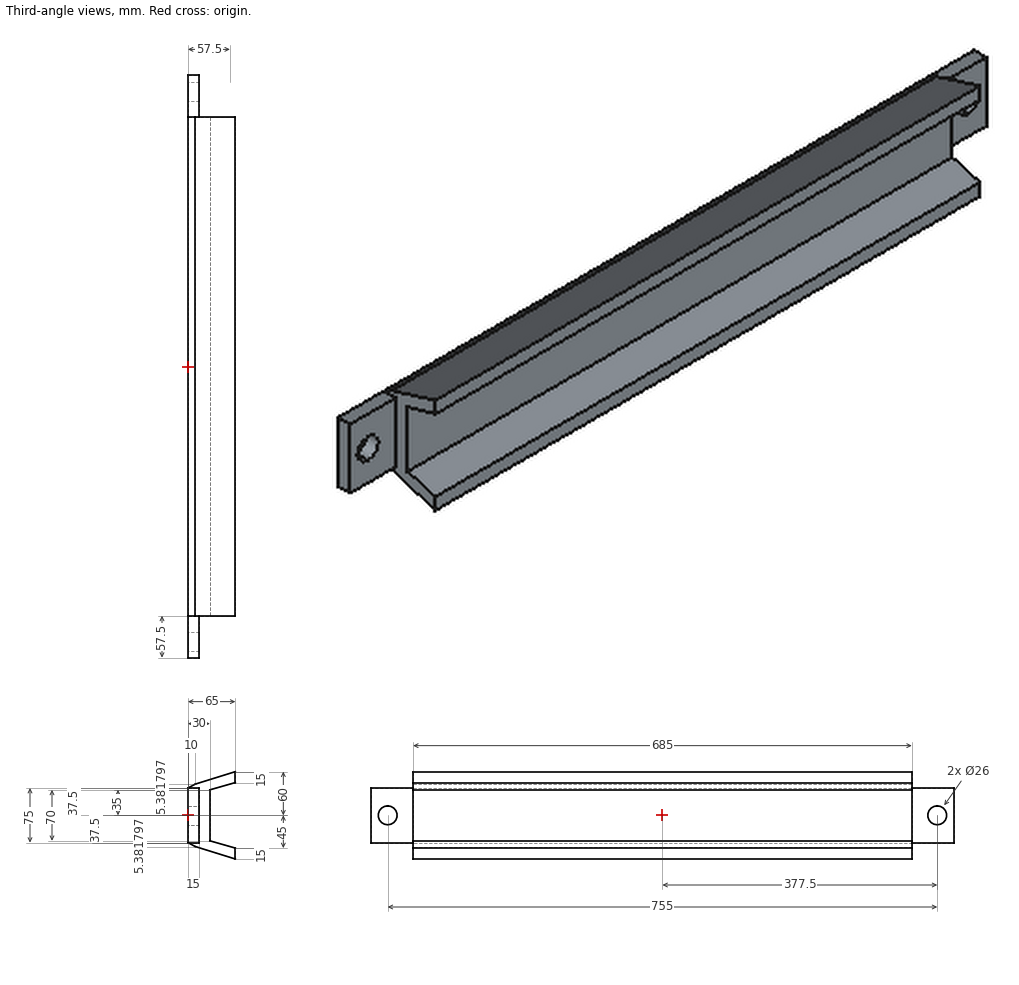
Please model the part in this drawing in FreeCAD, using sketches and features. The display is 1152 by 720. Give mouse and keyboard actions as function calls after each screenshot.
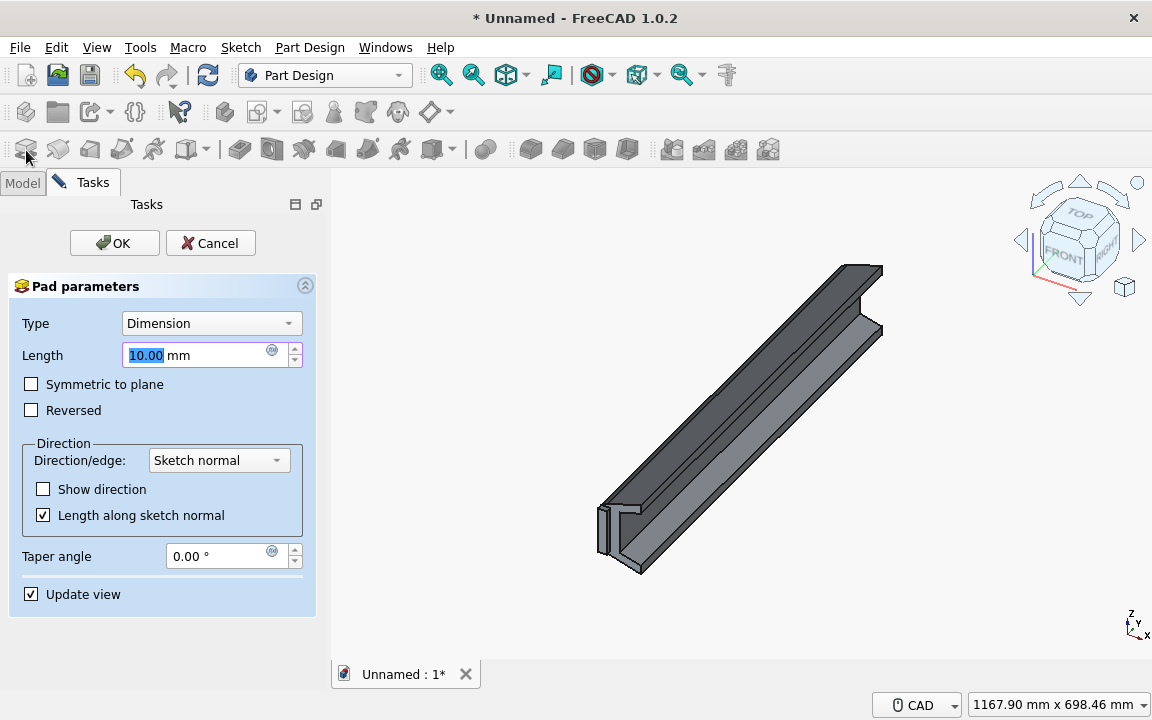
text(57.5)
key(Tab)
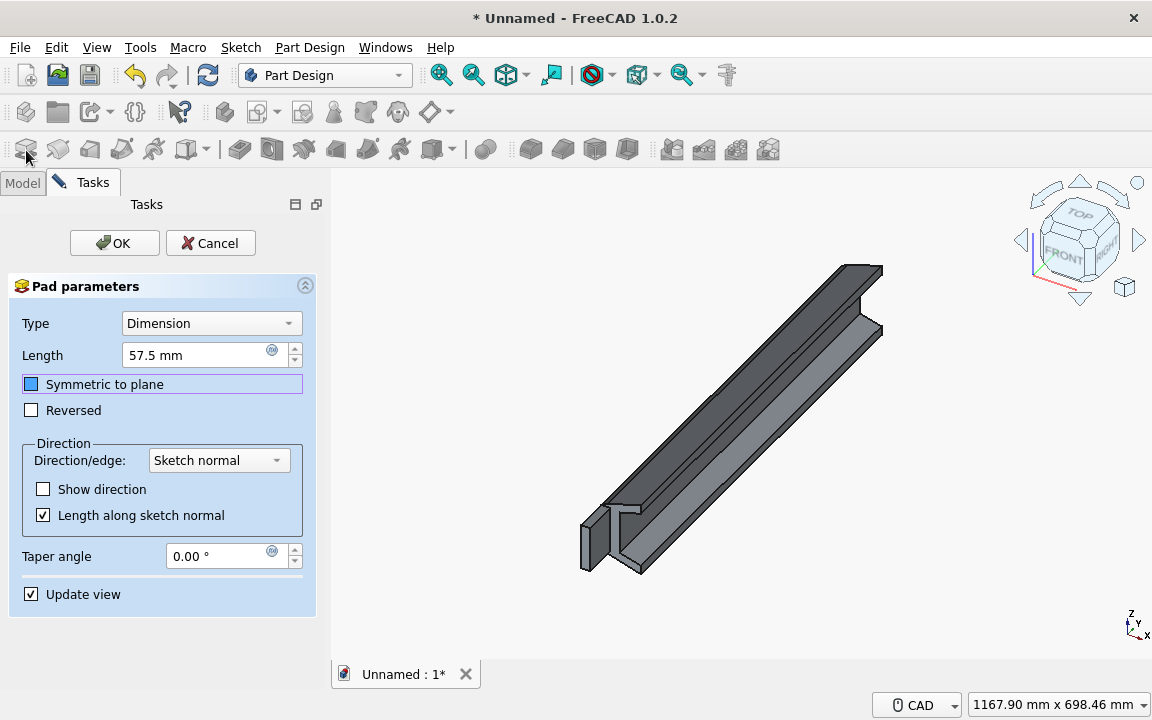
click(115, 243)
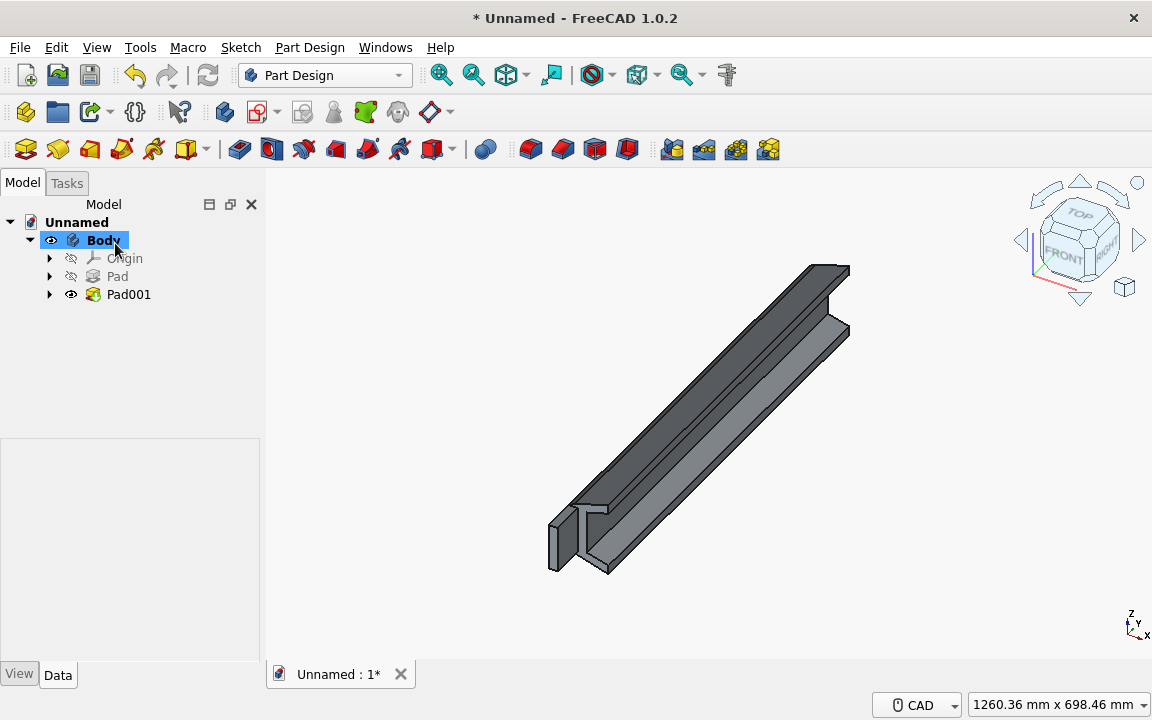
click(116, 294)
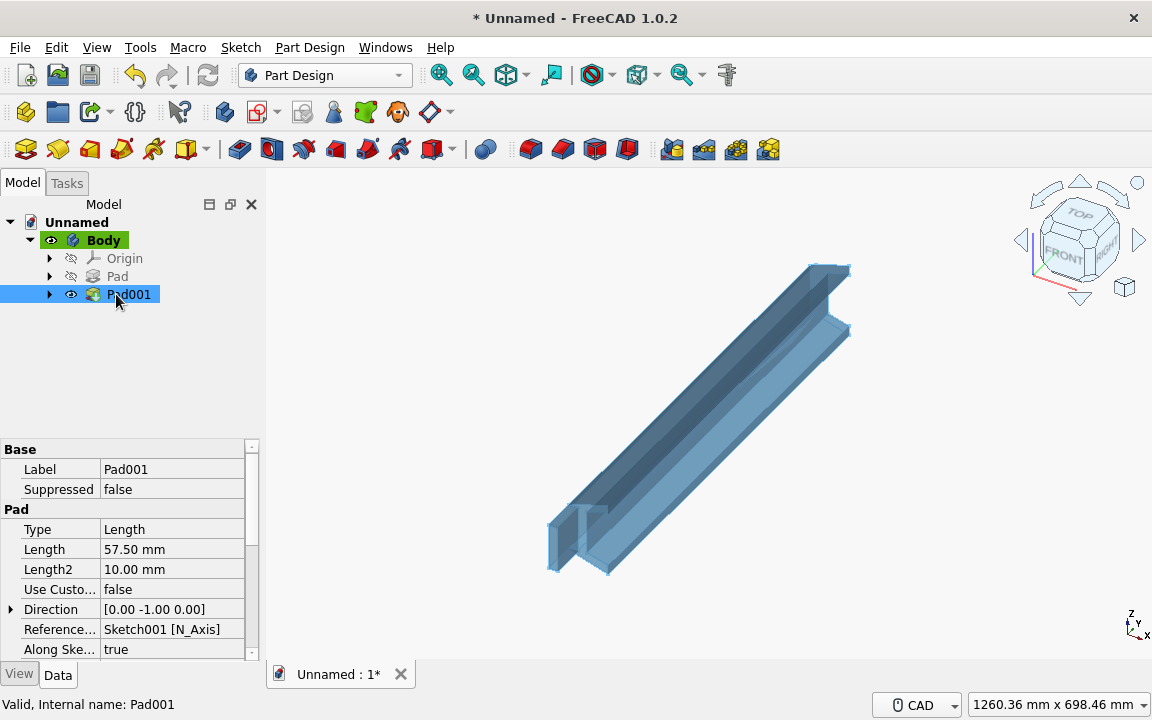
click(672, 150)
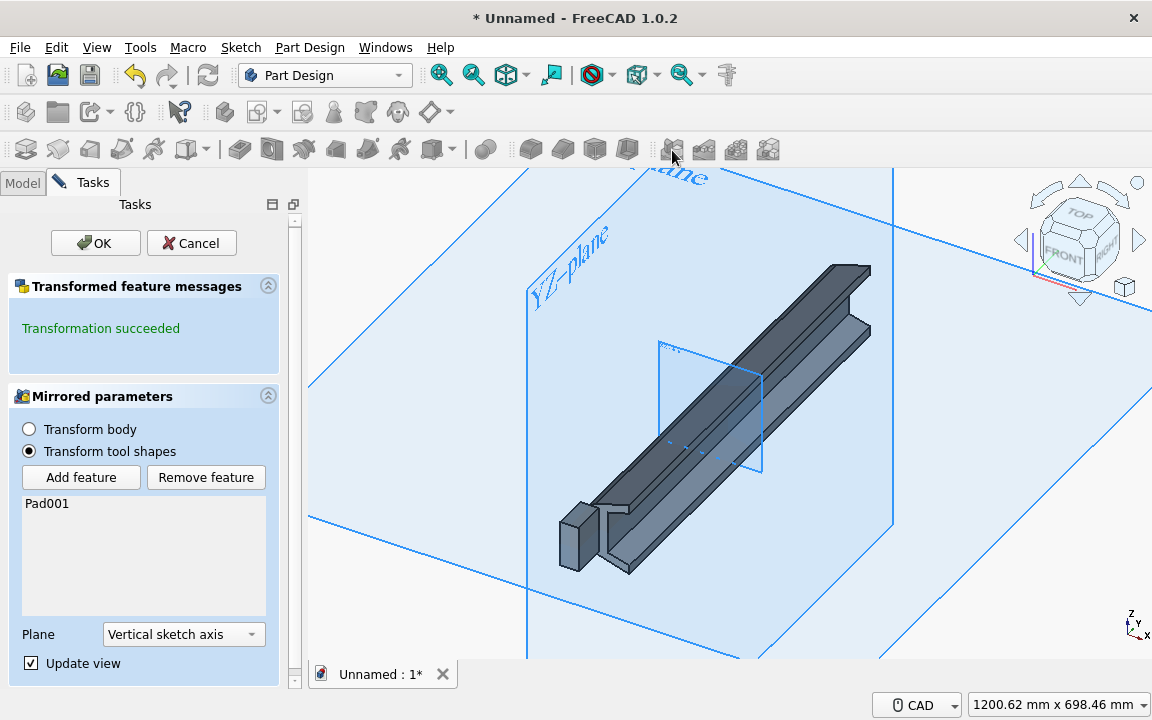
click(184, 634)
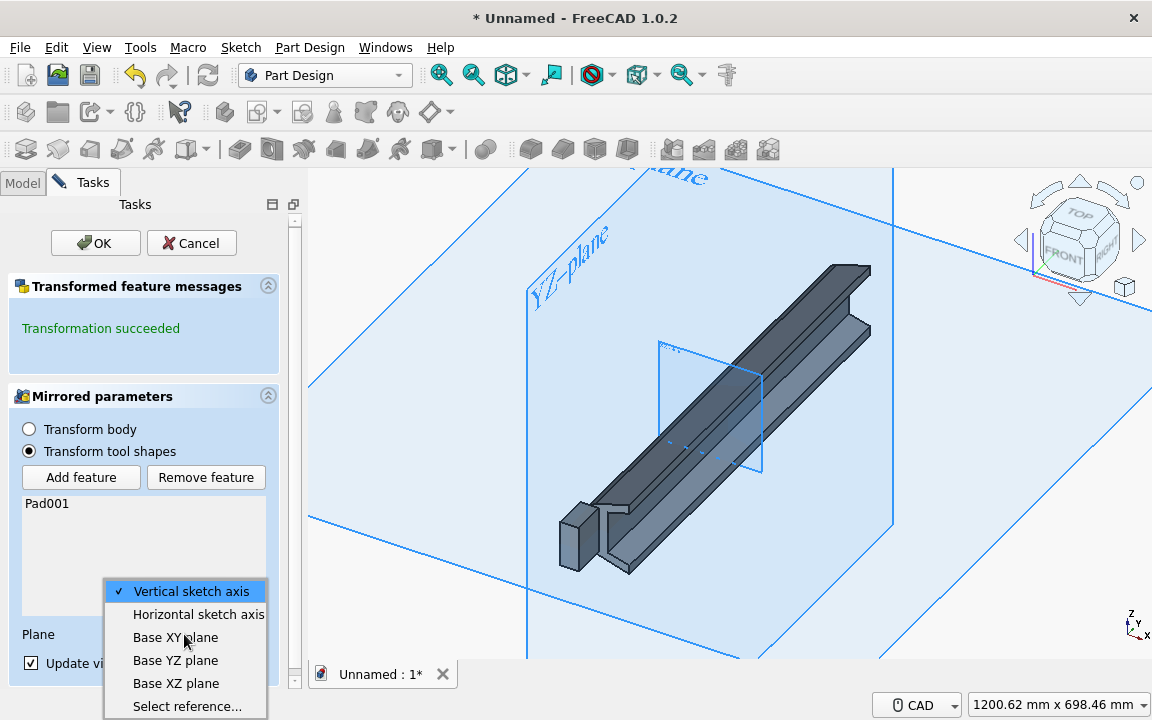
click(184, 684)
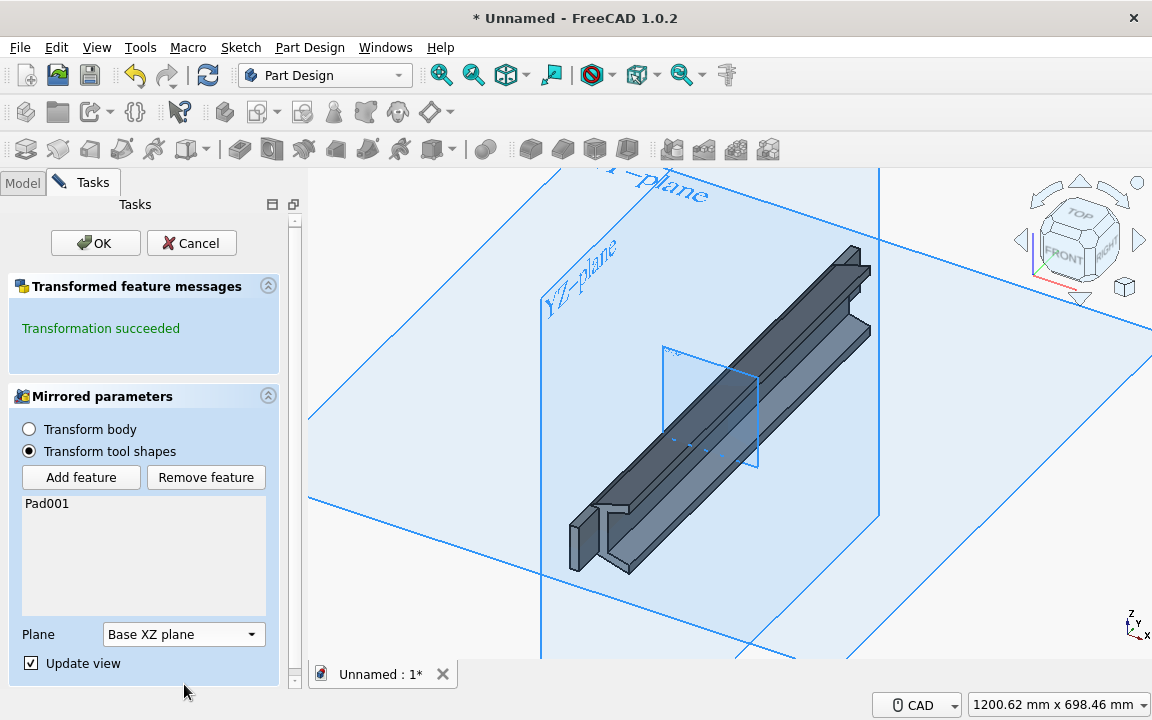
click(96, 243)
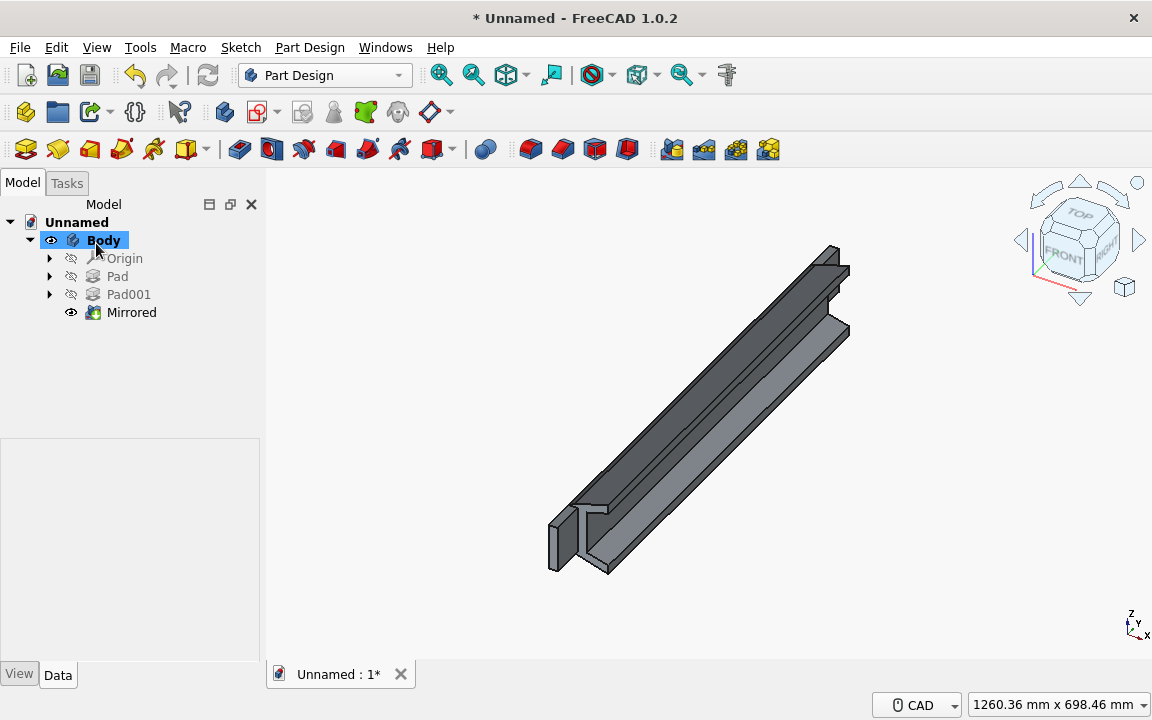
key(6)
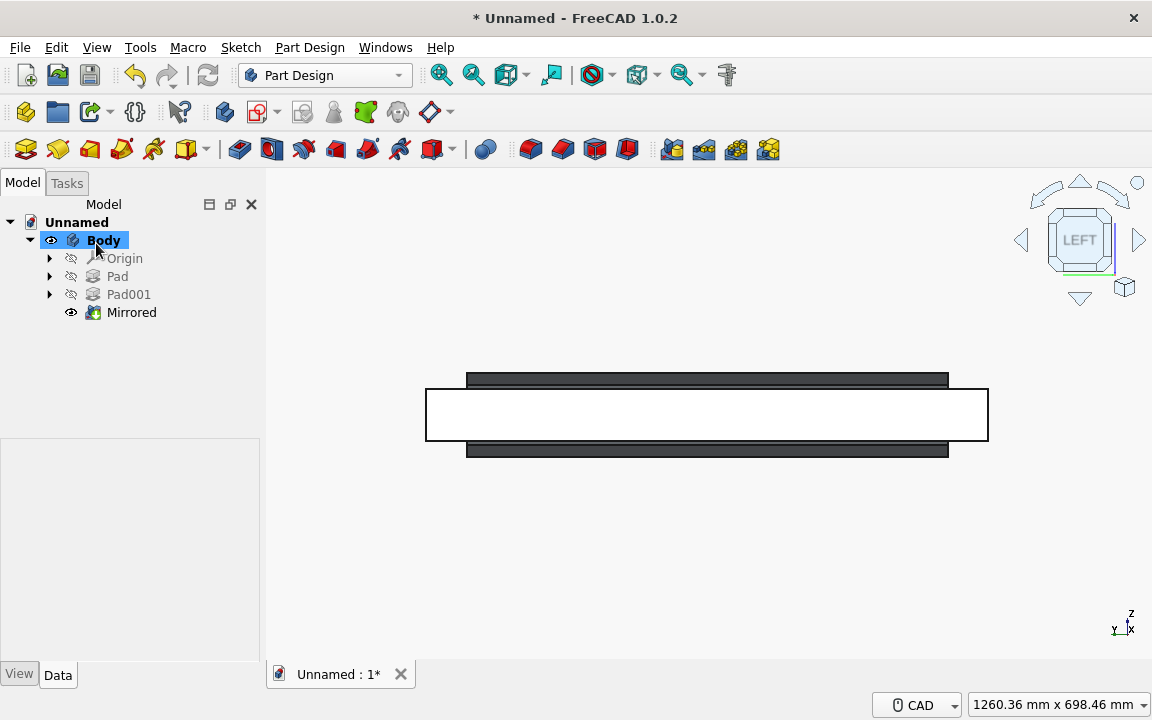
click(707, 414)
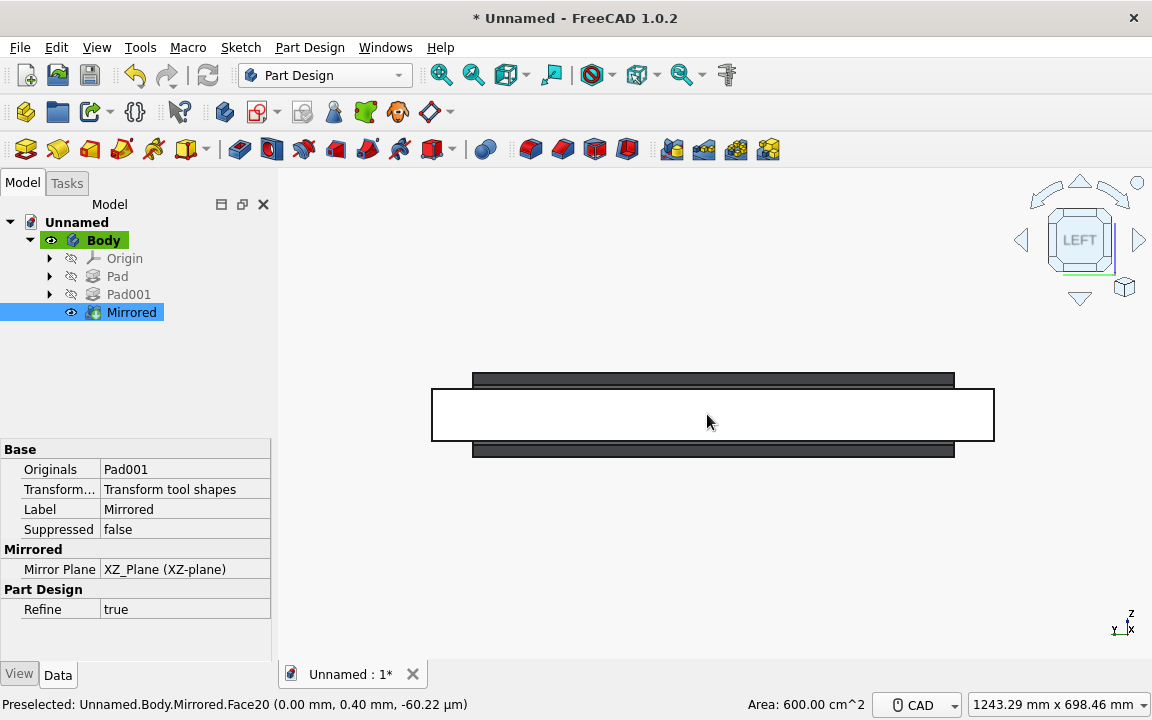
click(258, 112)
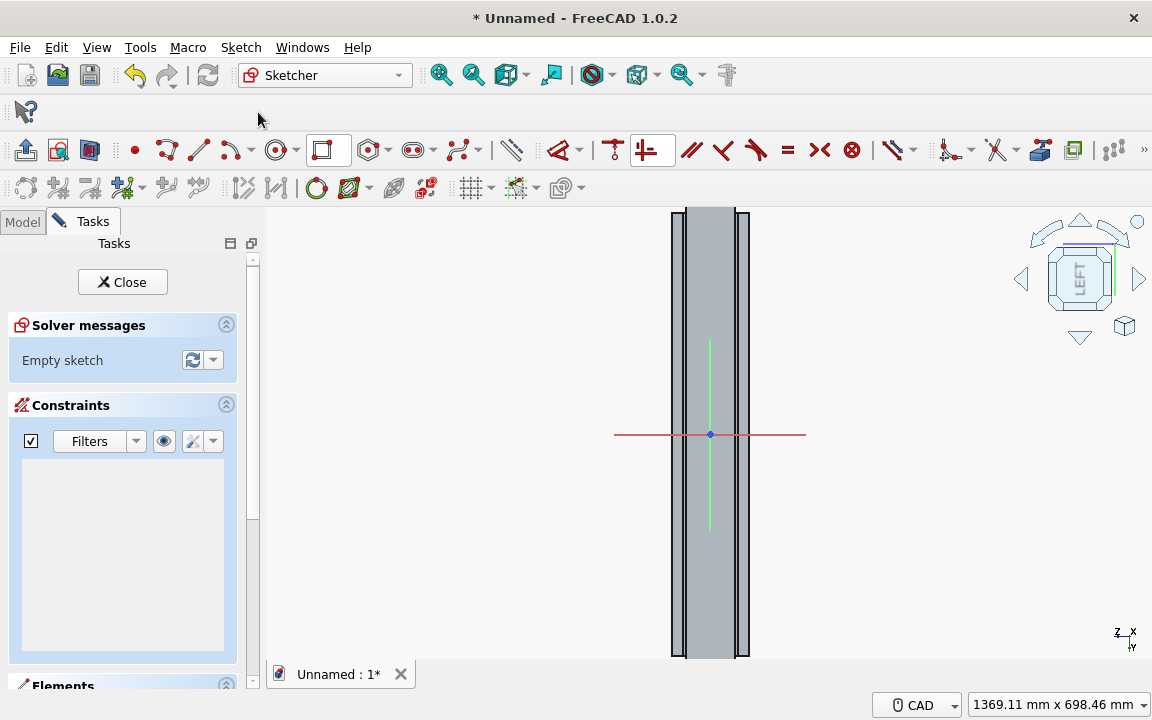
scroll(556, 431, down, 3)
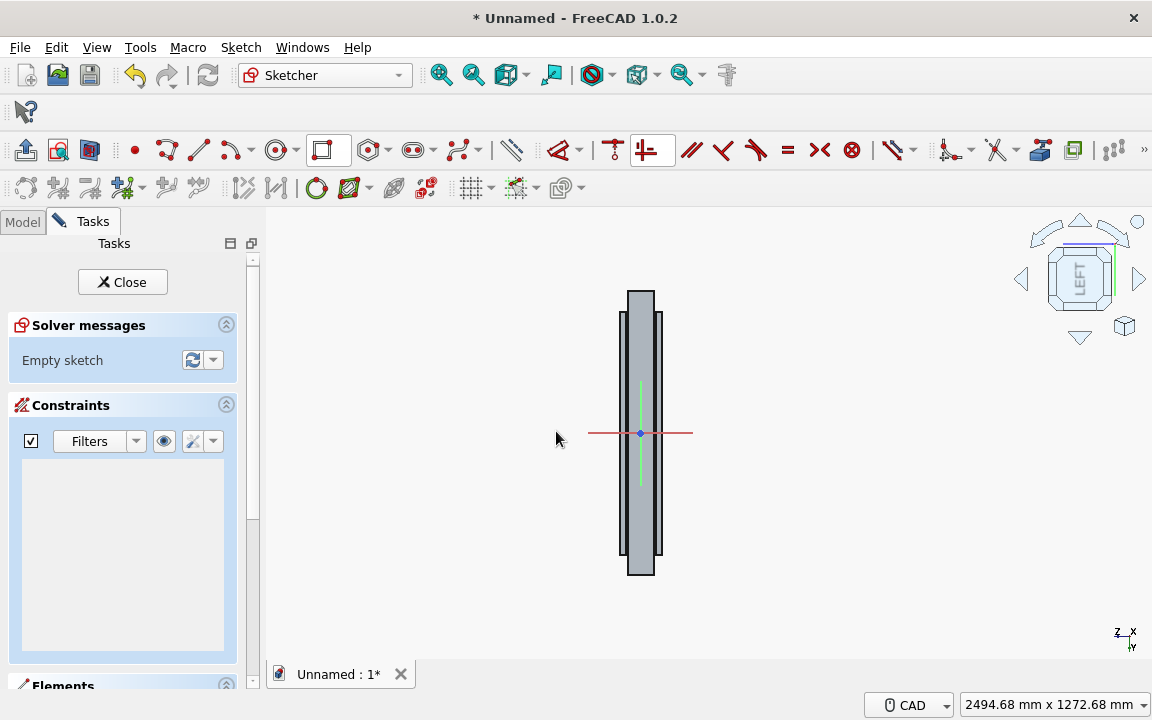
click(276, 150)